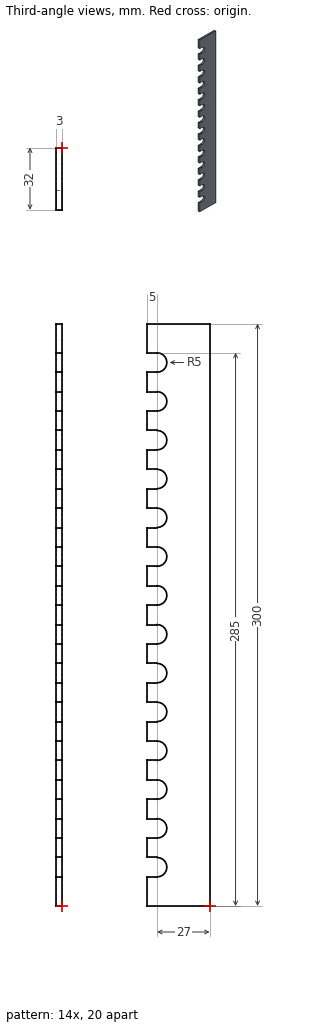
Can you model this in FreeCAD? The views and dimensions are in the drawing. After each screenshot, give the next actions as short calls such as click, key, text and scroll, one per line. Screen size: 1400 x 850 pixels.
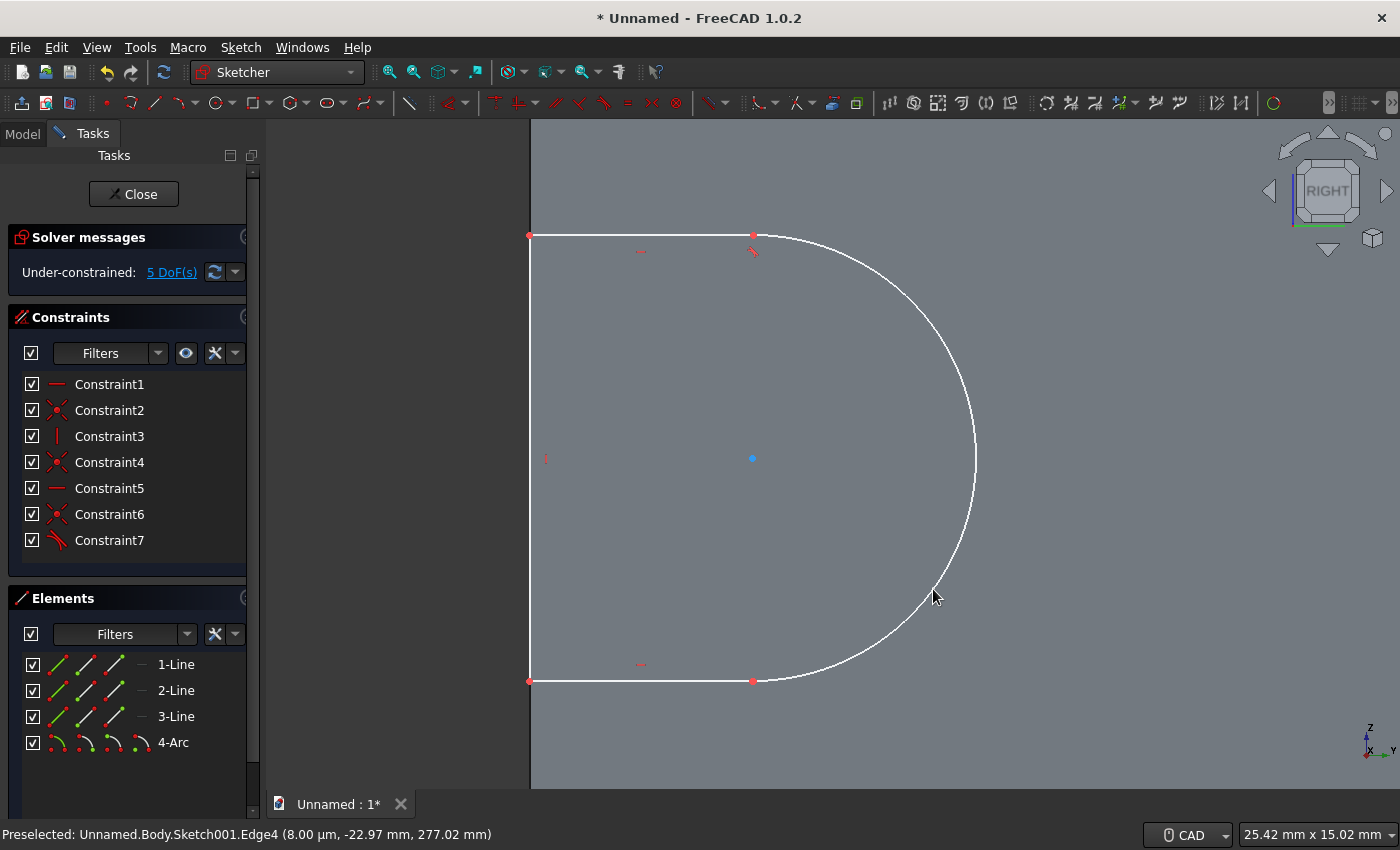
click(597, 681)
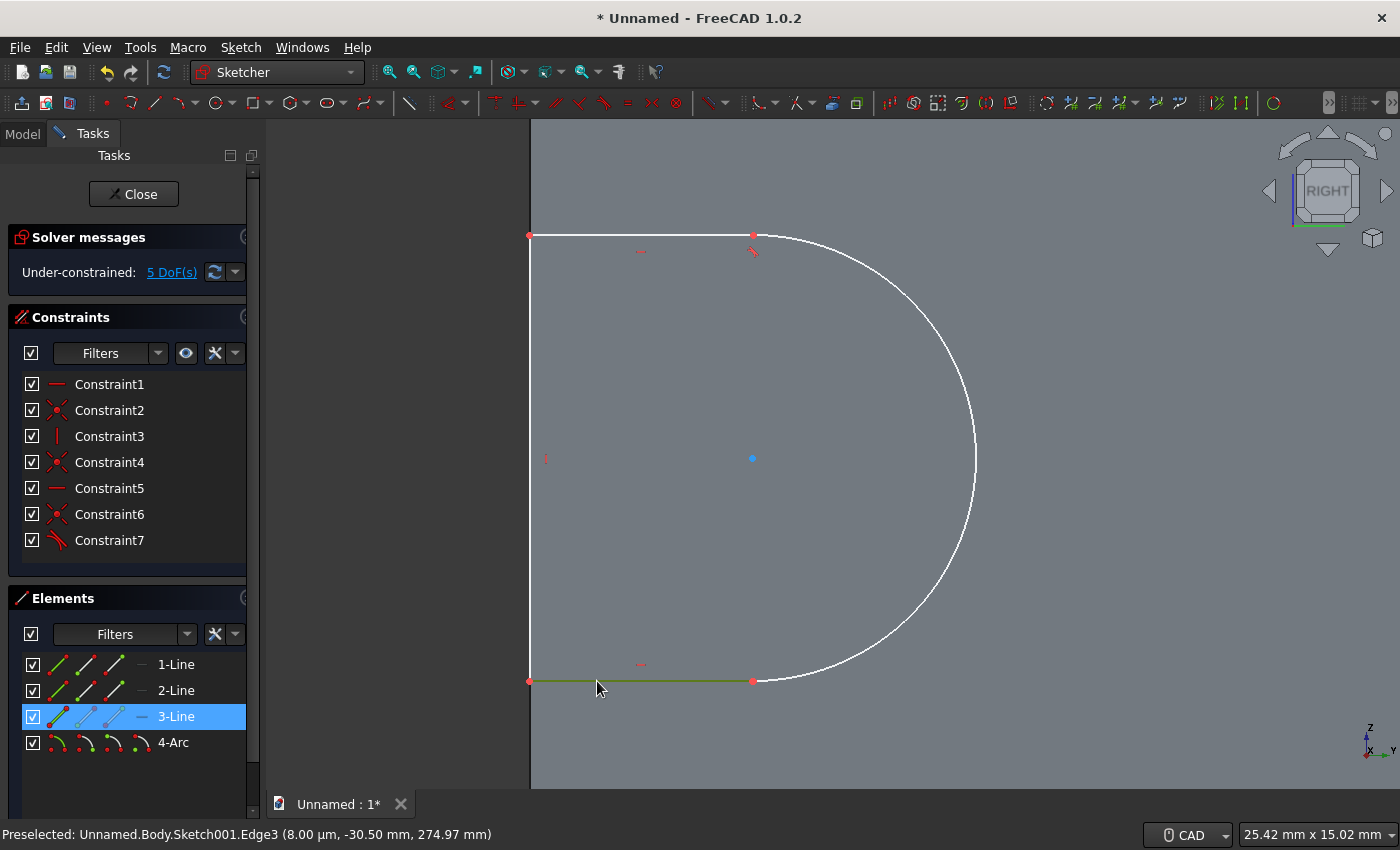
click(933, 589)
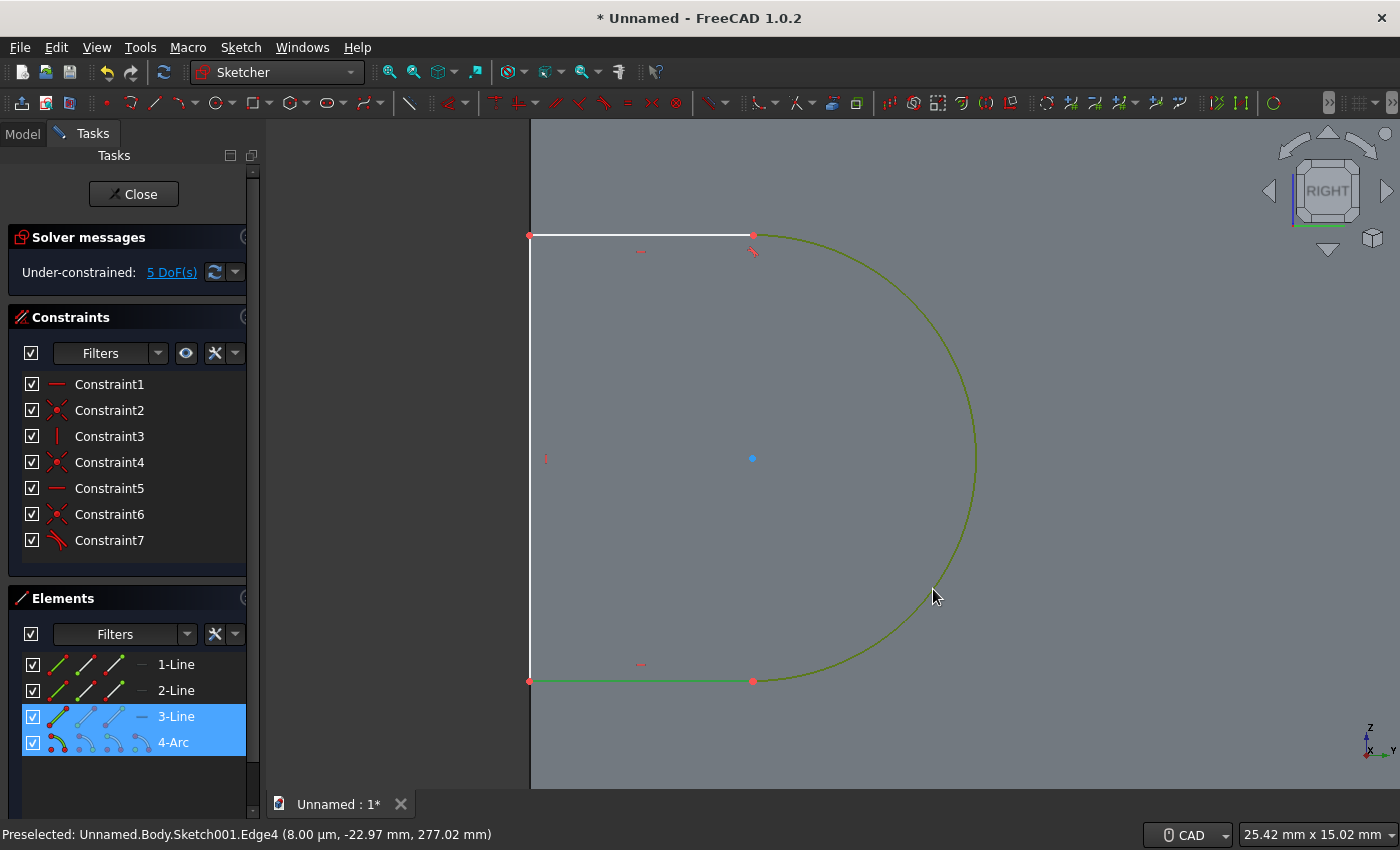
key(t)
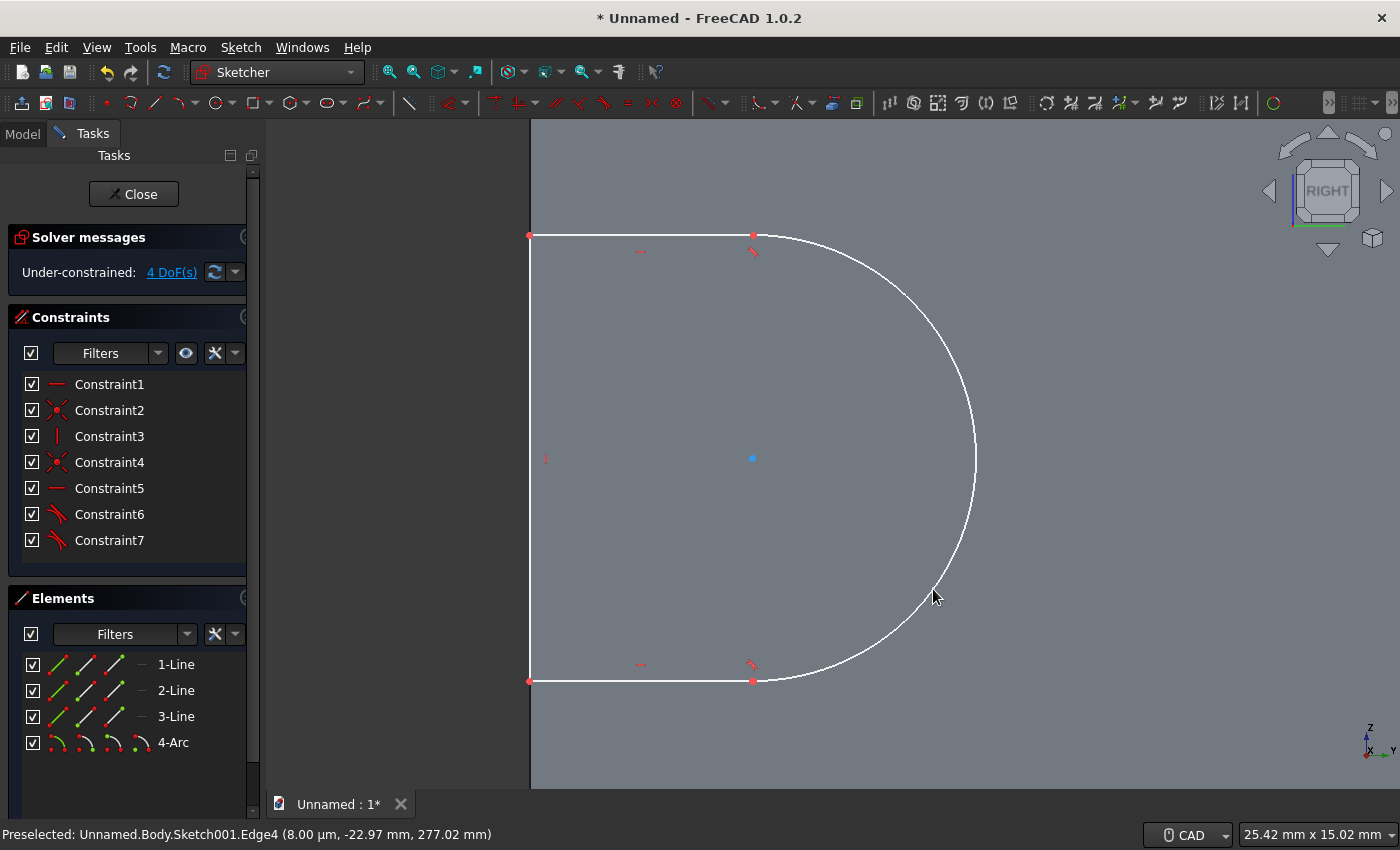
key(d)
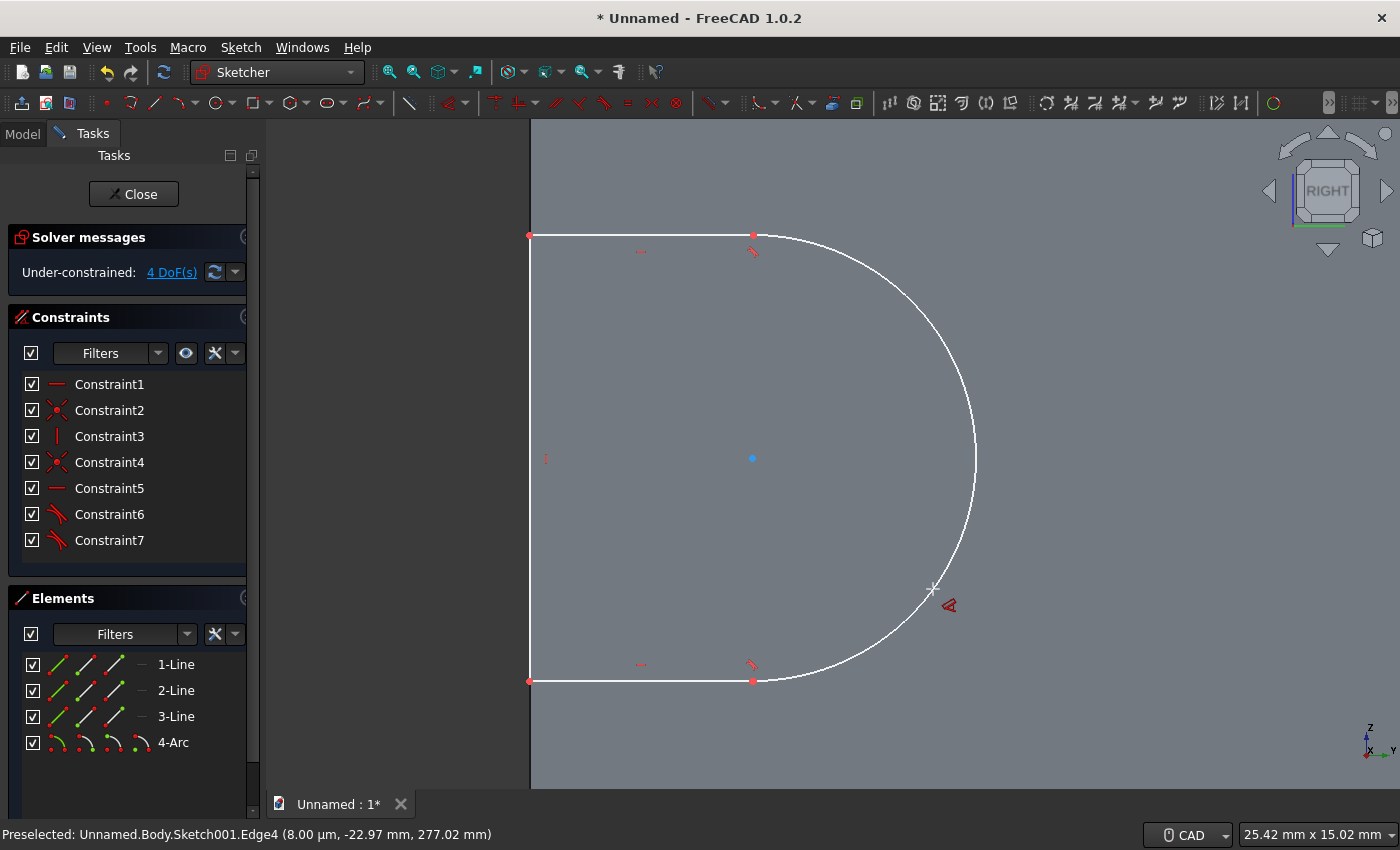
click(933, 589)
click(959, 608)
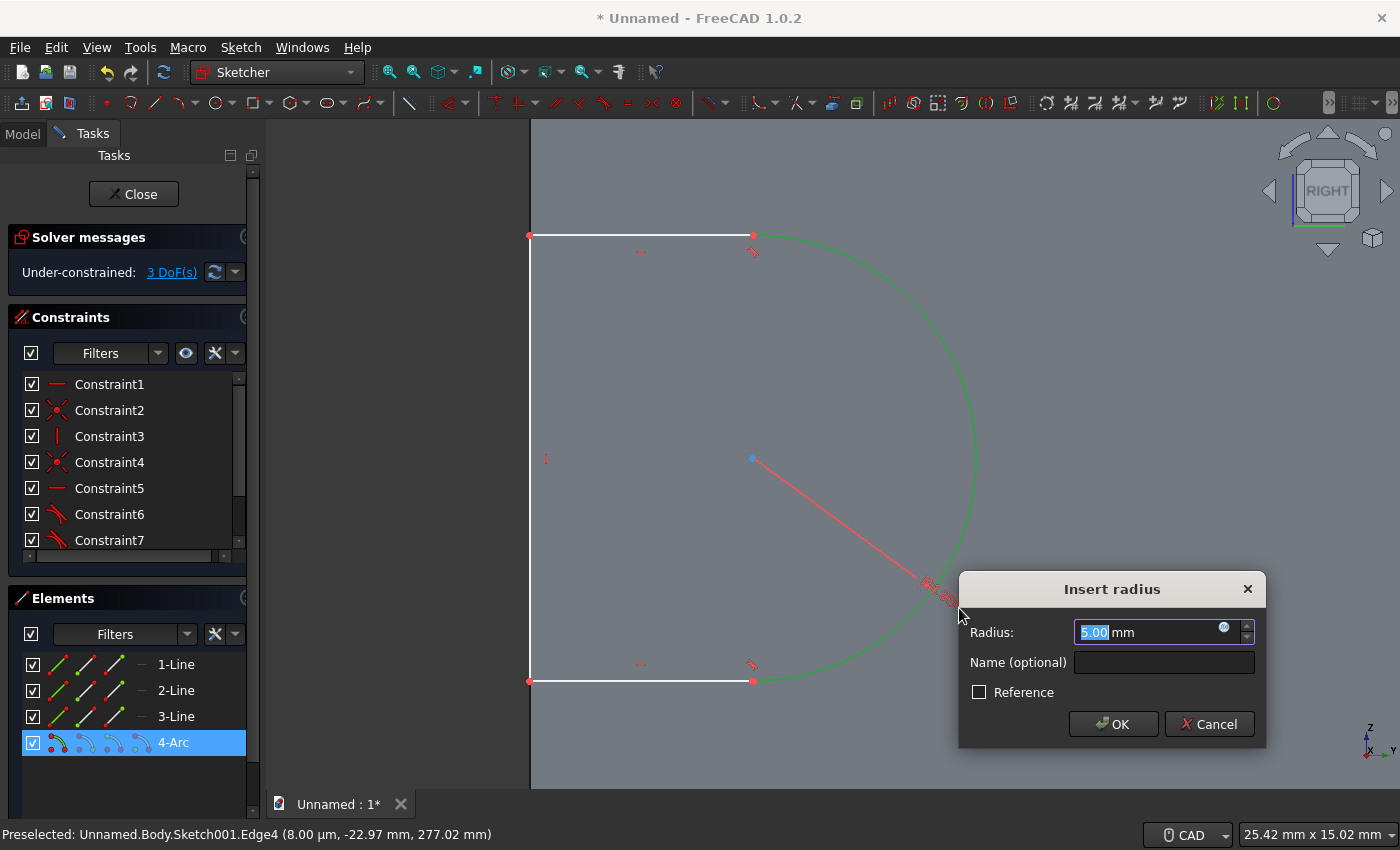
text(5)
key(Return)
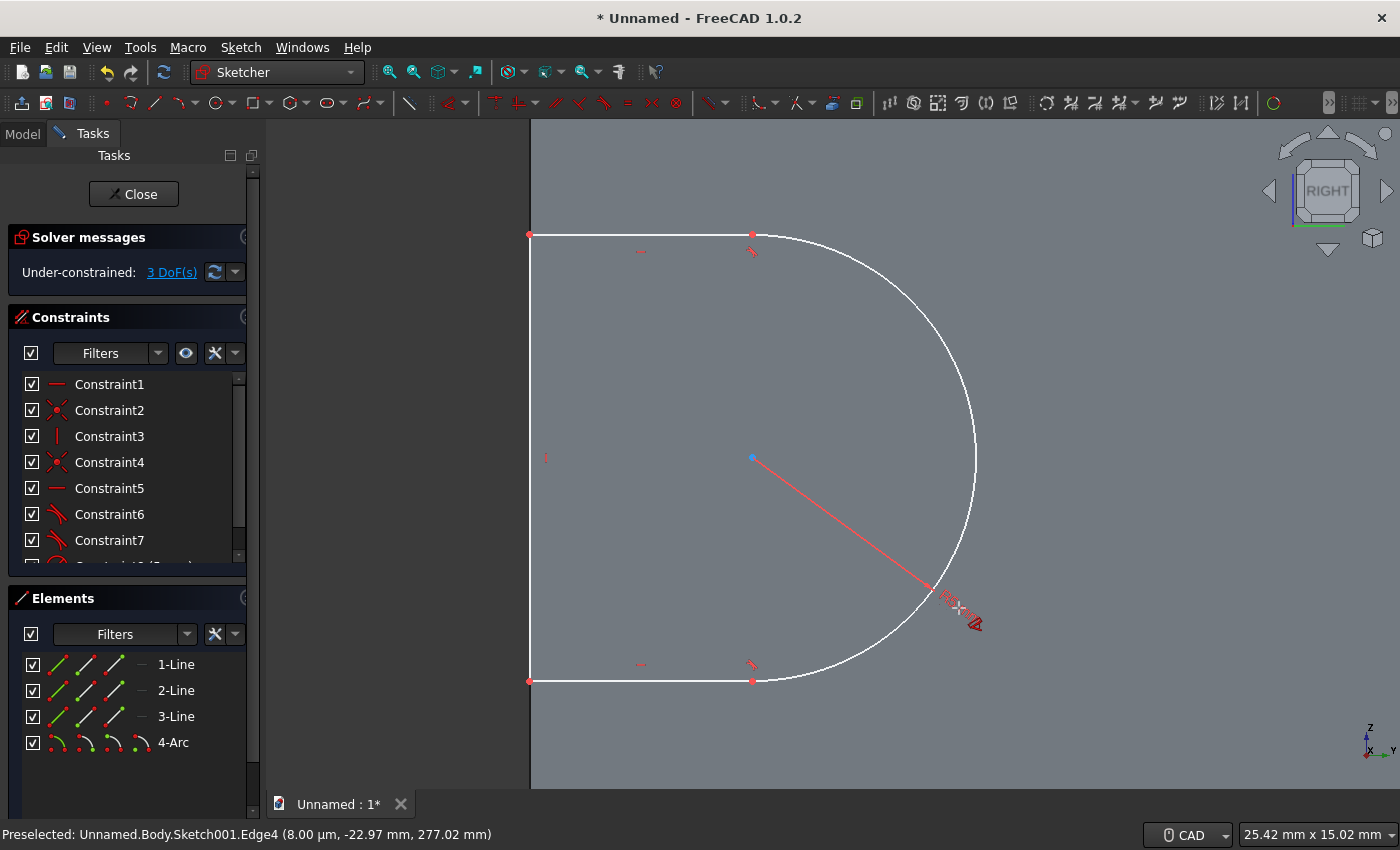
click(686, 235)
click(641, 201)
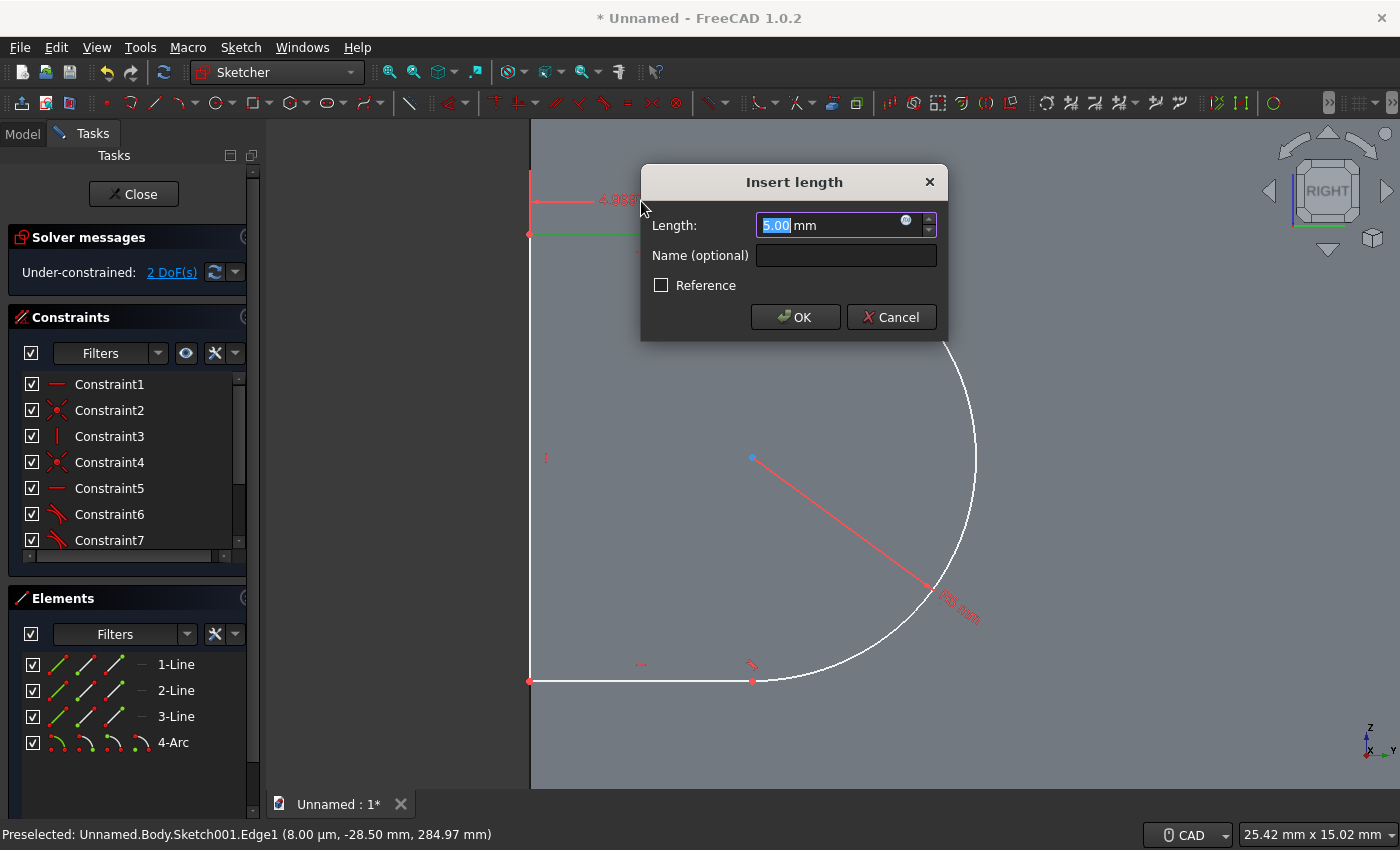
text(5)
key(Return)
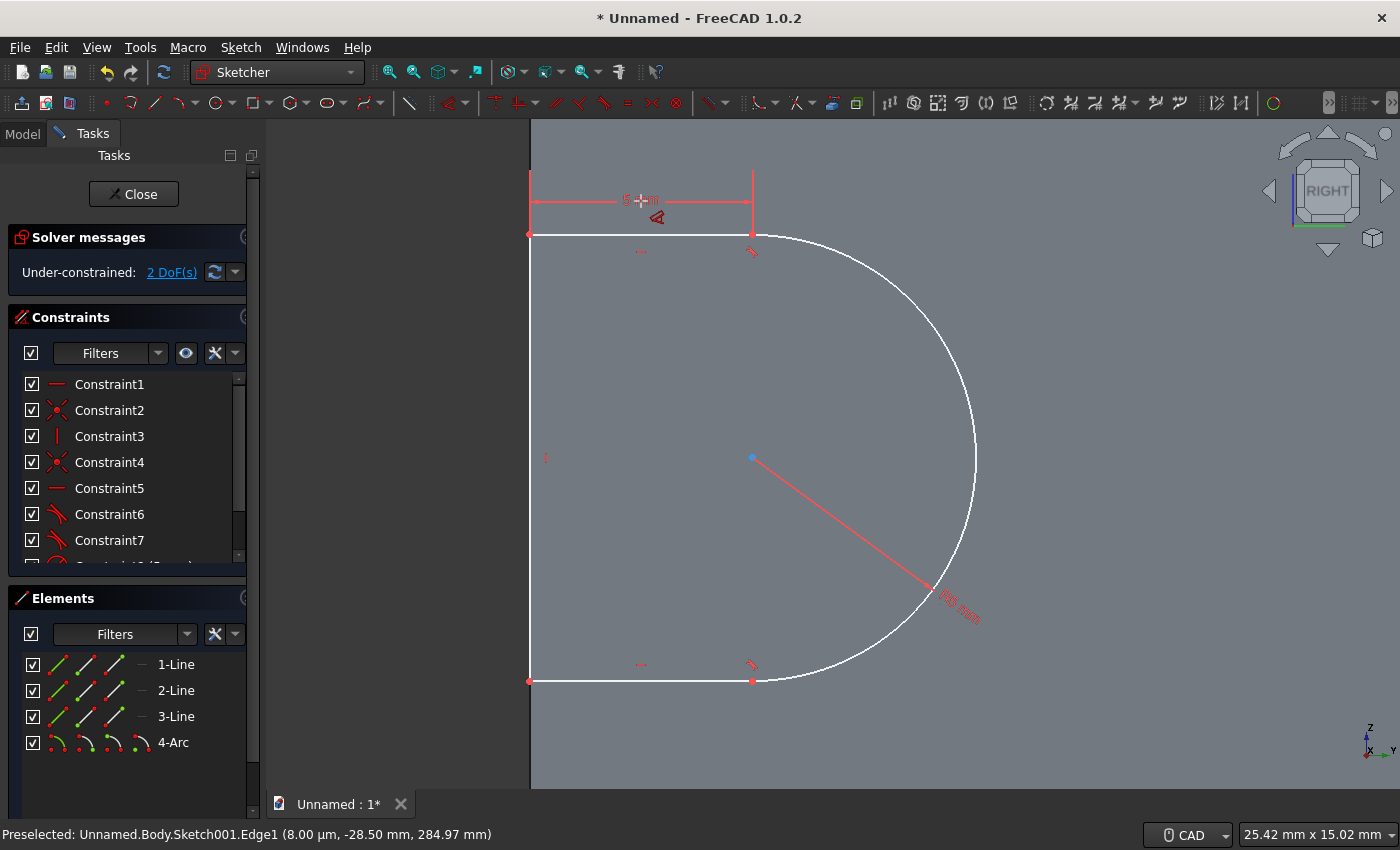
click(753, 235)
click(994, 201)